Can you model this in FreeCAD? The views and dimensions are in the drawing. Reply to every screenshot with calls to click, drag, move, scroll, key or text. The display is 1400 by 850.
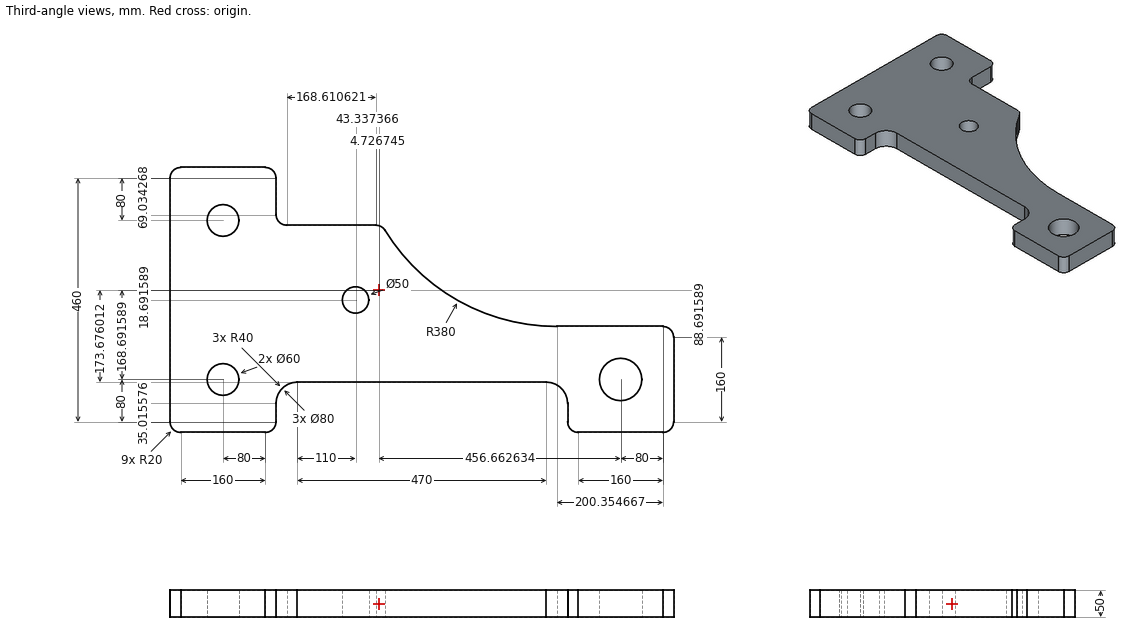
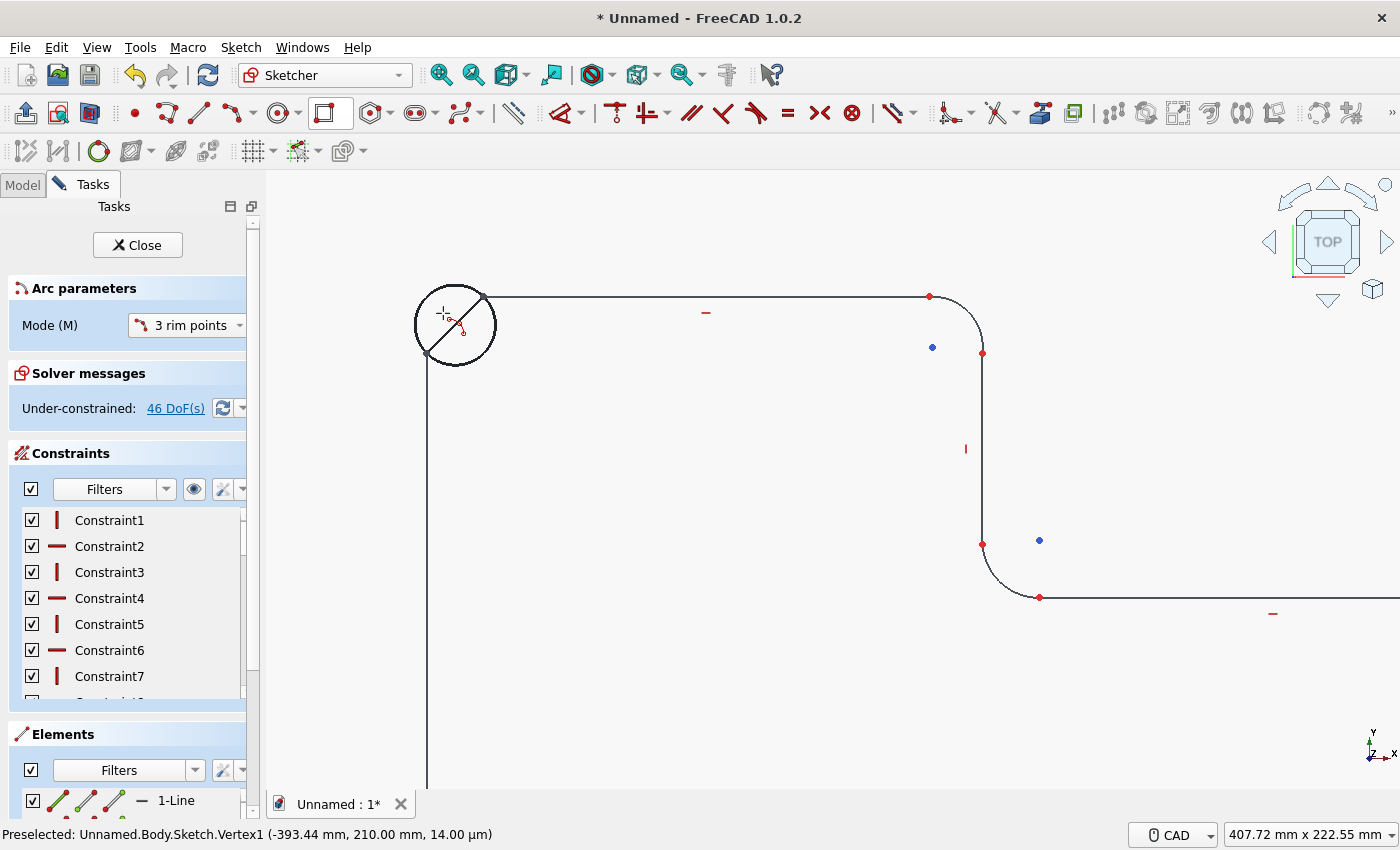
click(443, 310)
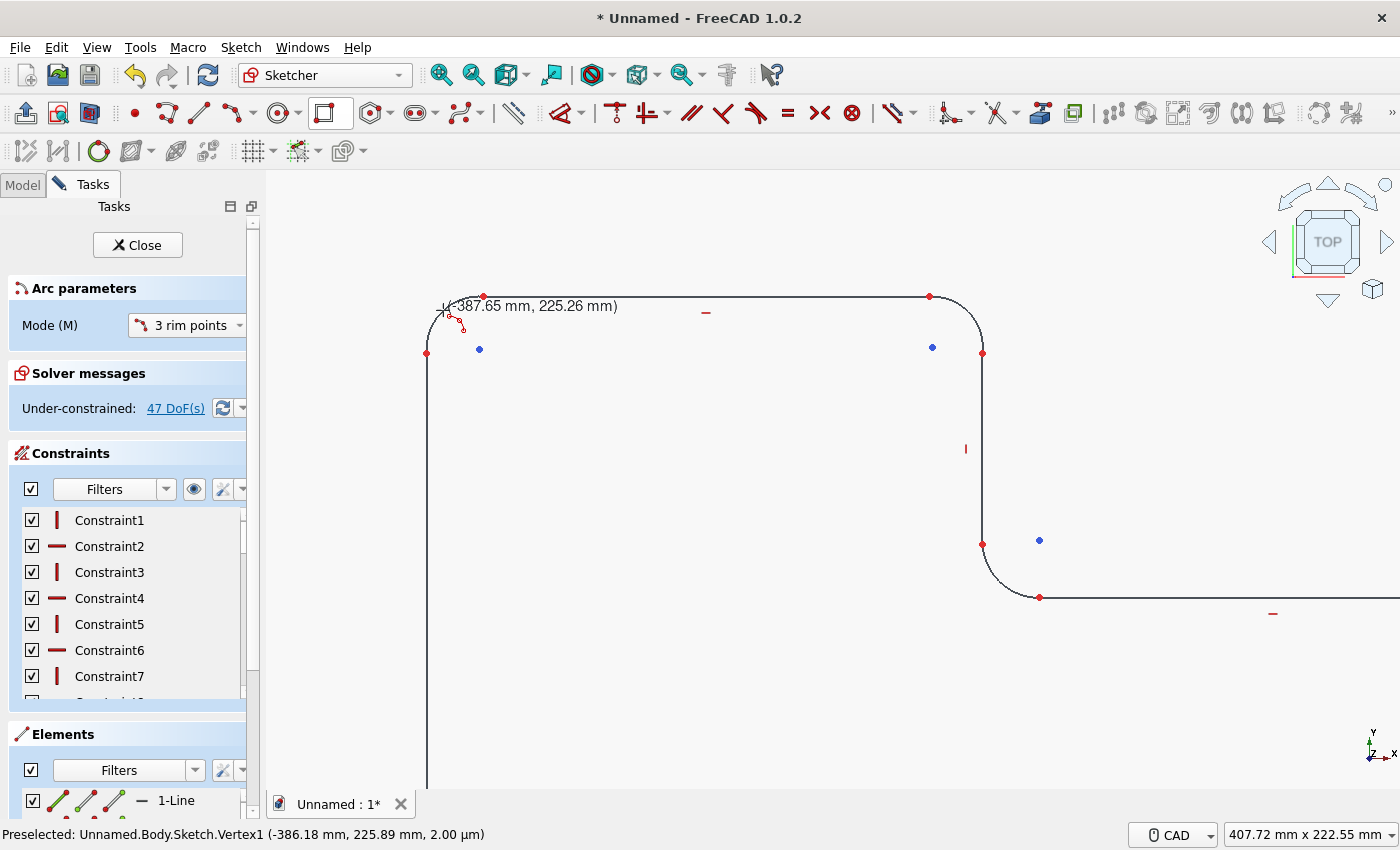
click(278, 114)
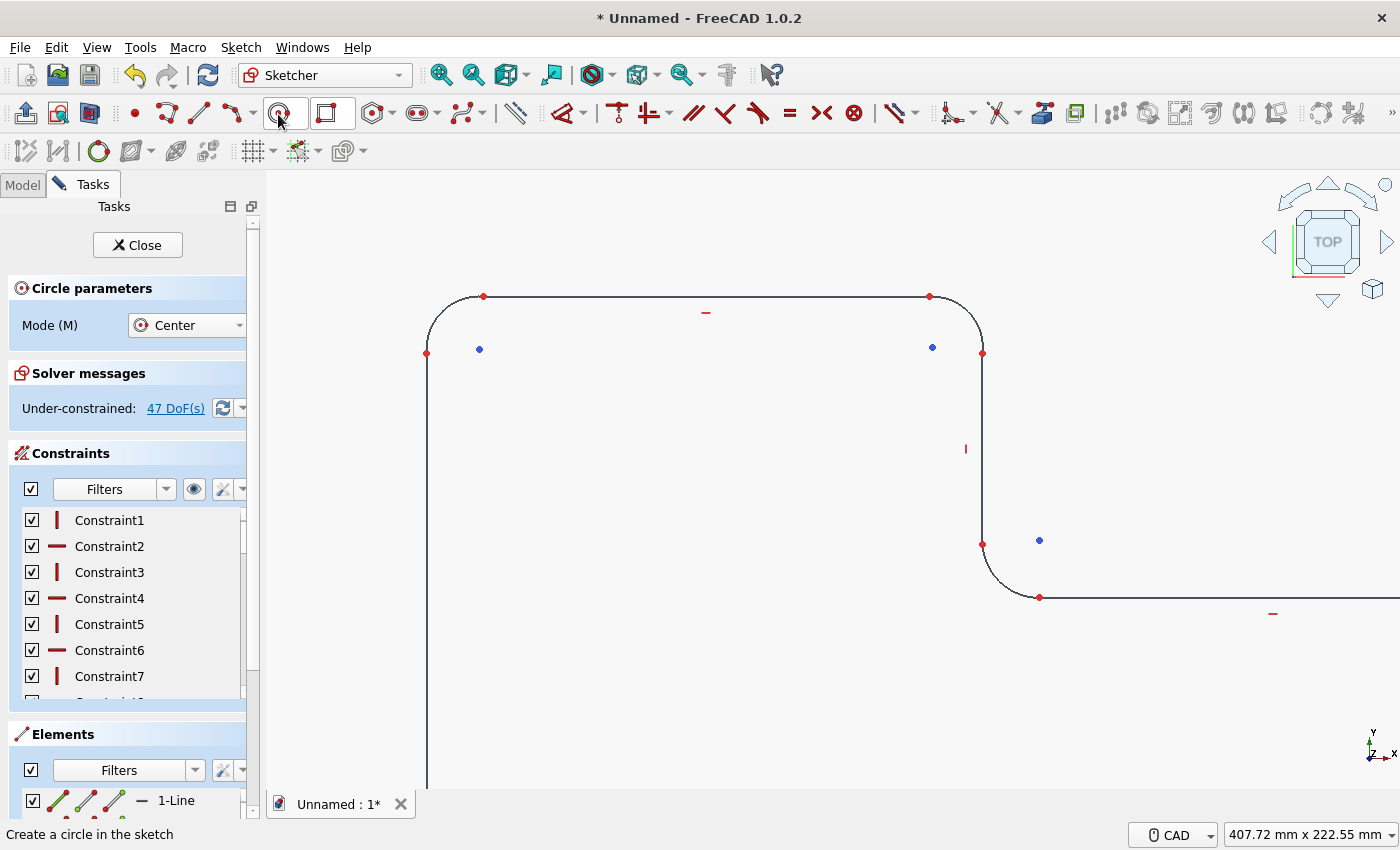
scroll(442, 313, down, 7)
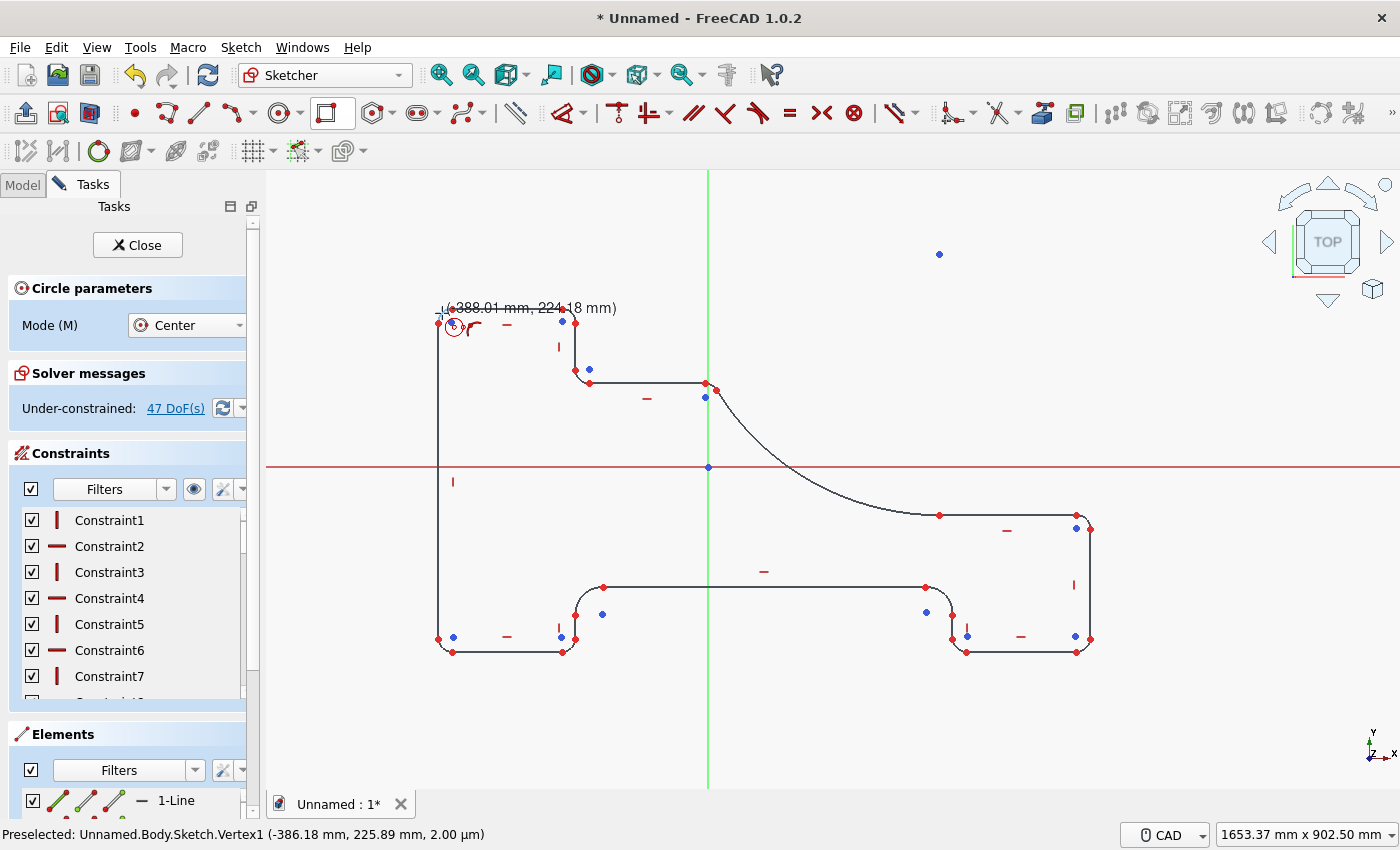
click(507, 583)
move(522, 568)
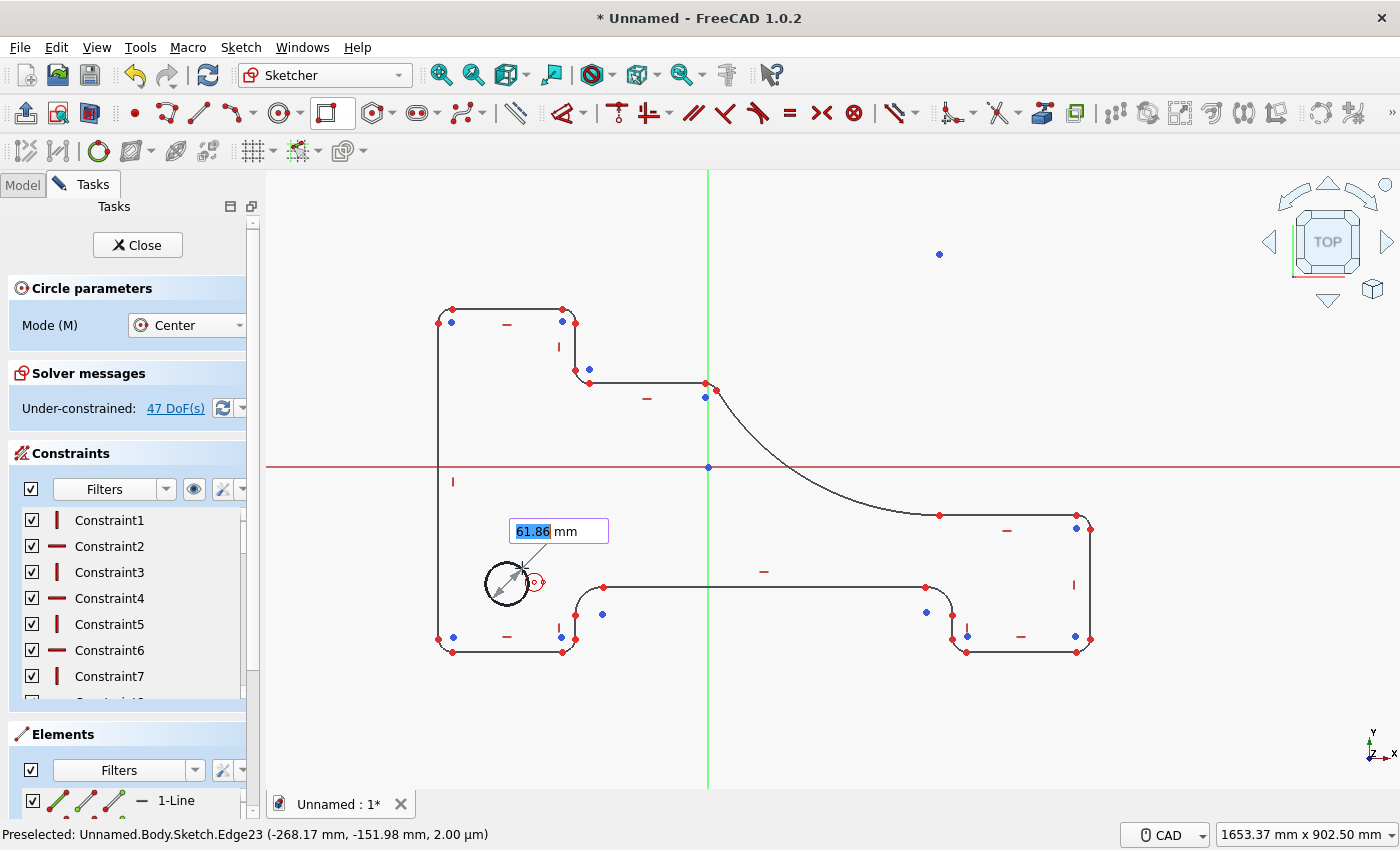
text(60)
key(Return)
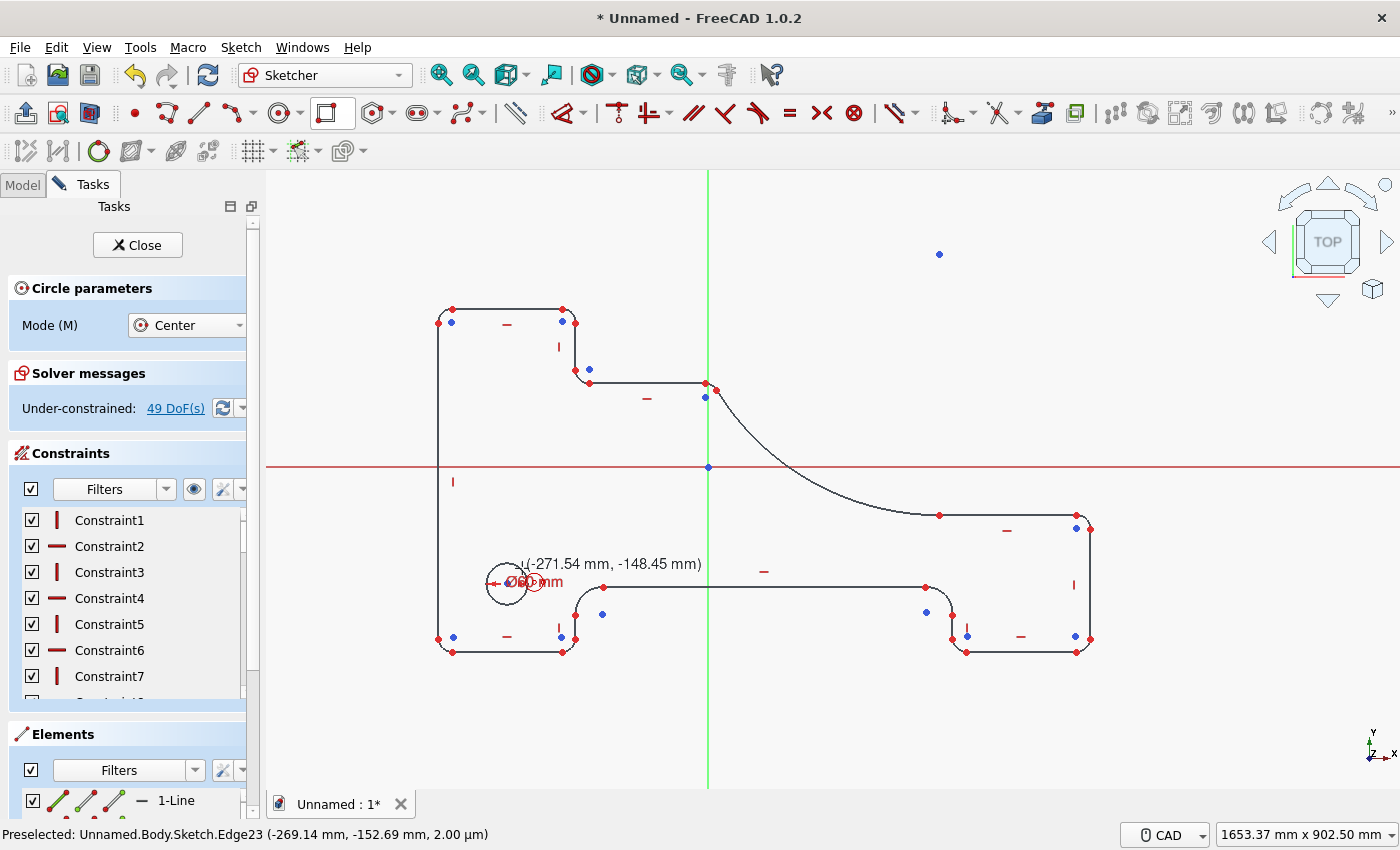
click(1021, 583)
move(1041, 563)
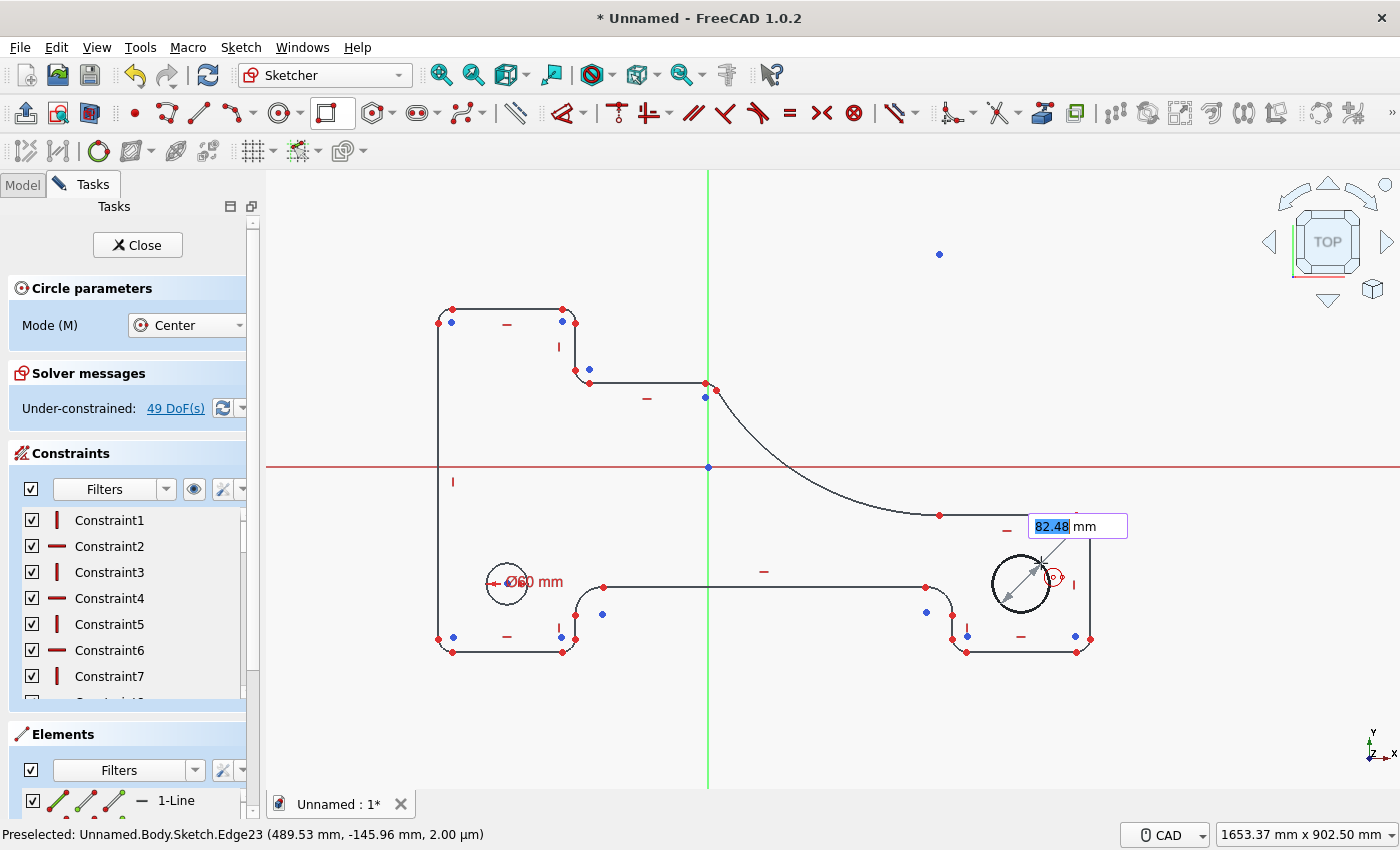
text(80)
key(Return)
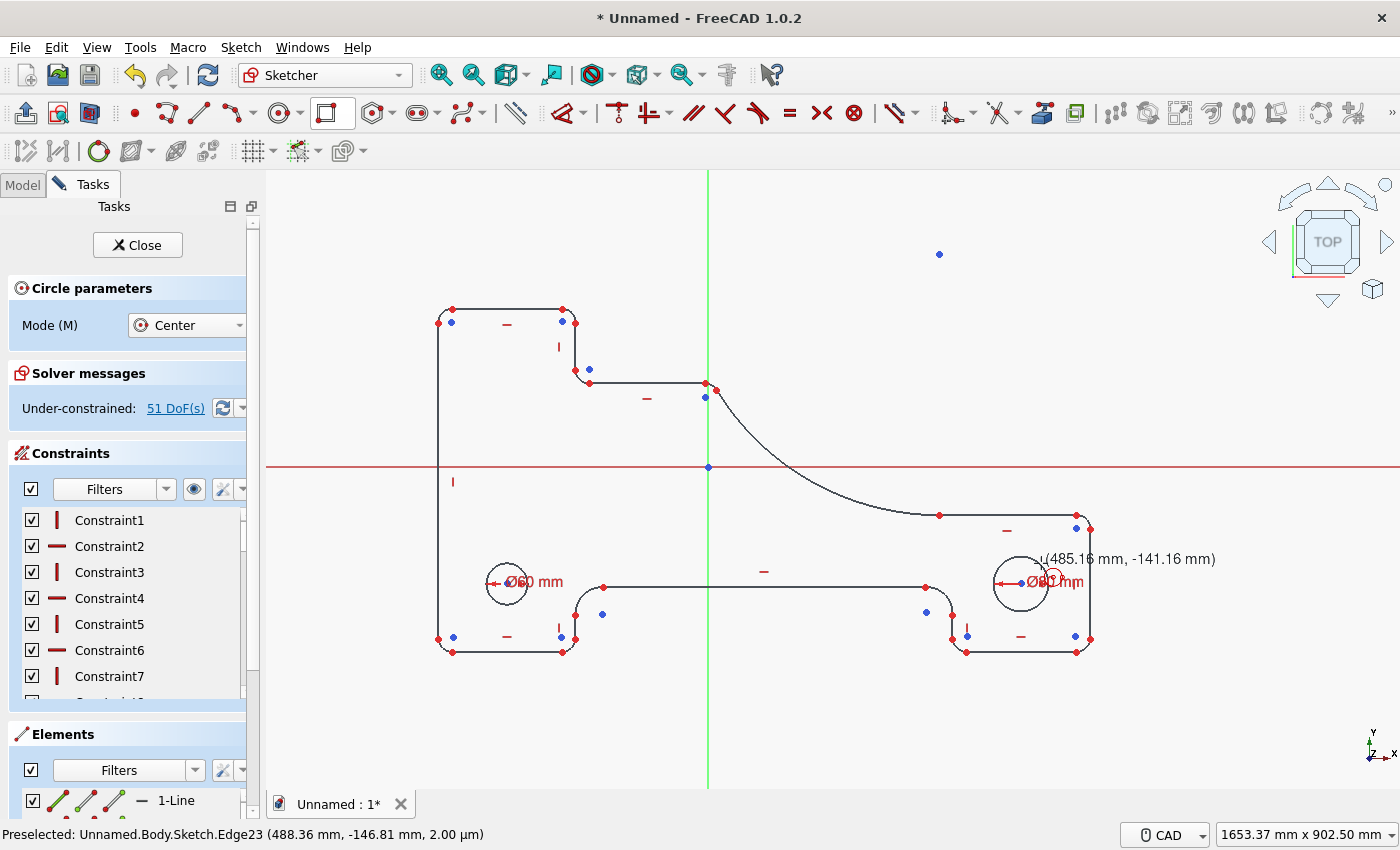
scroll(679, 480, up, 2)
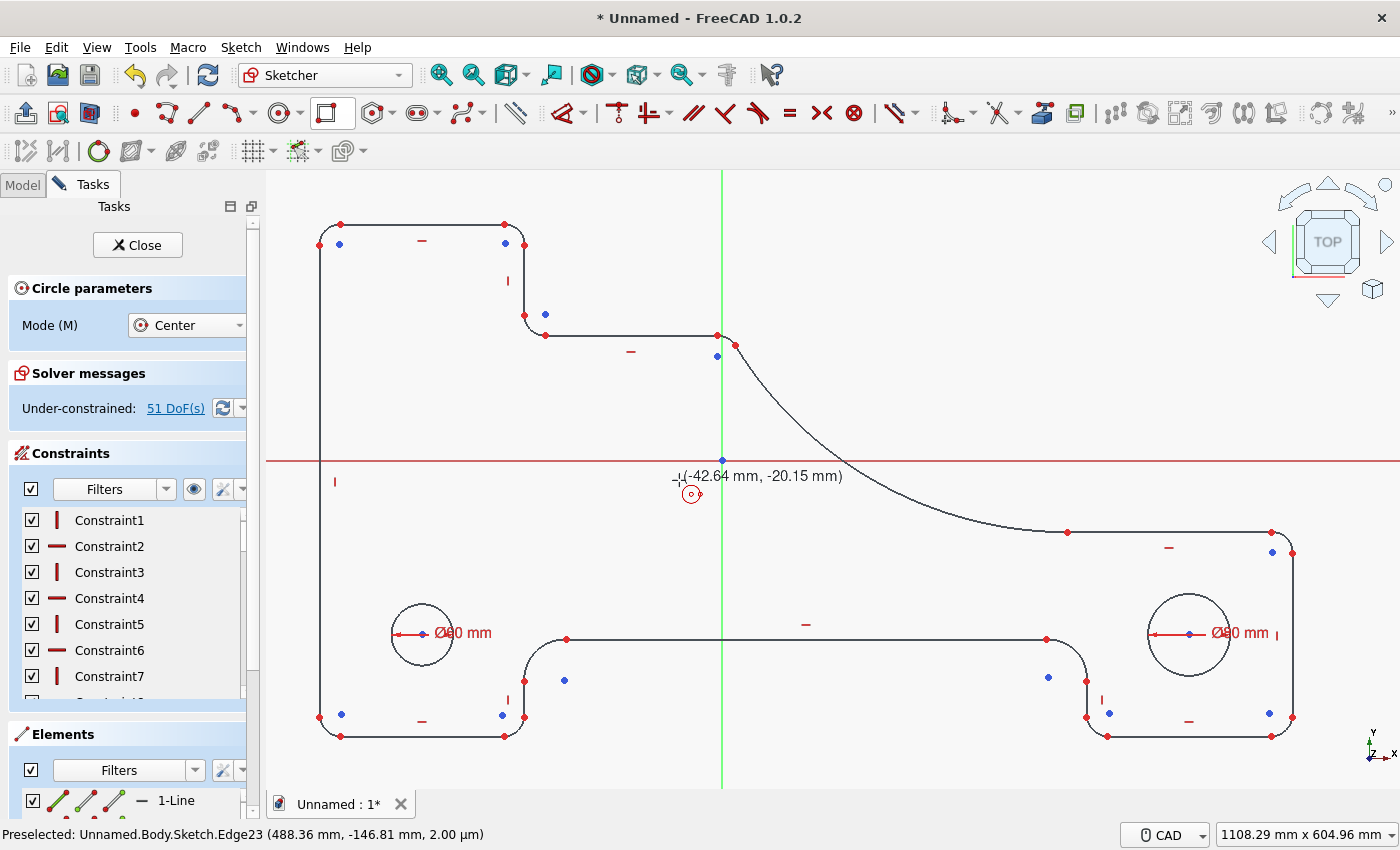
click(678, 480)
move(696, 498)